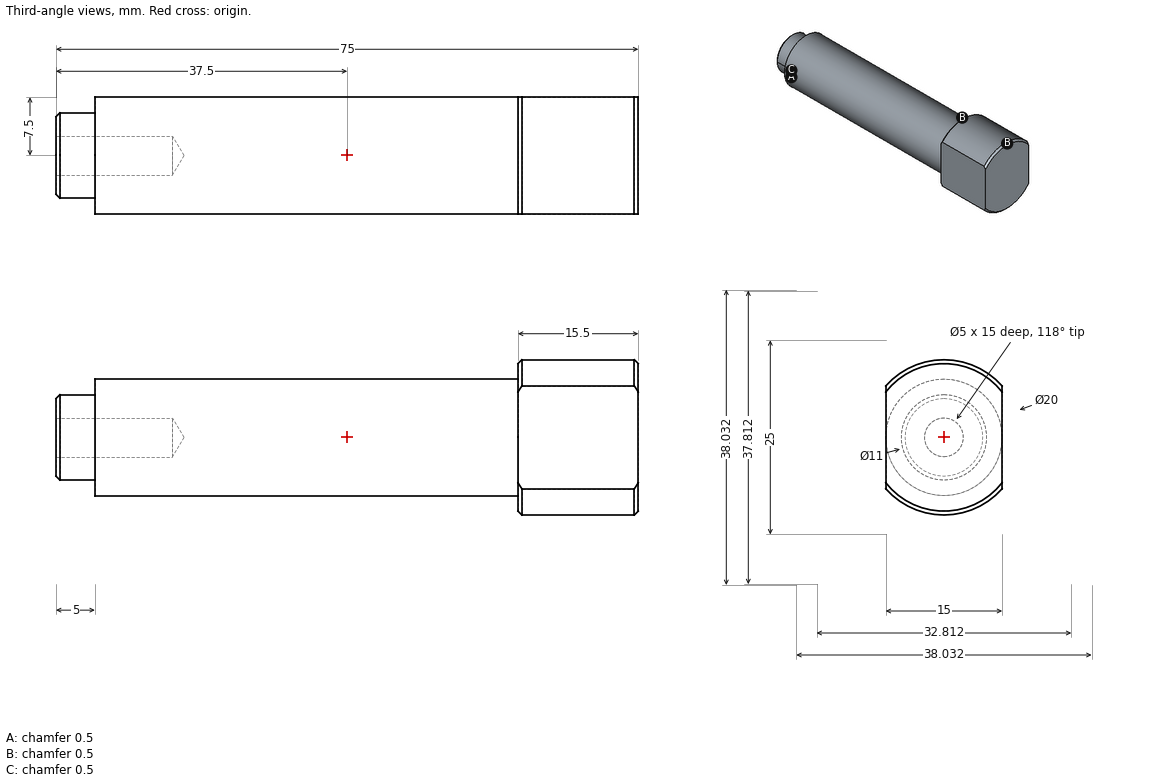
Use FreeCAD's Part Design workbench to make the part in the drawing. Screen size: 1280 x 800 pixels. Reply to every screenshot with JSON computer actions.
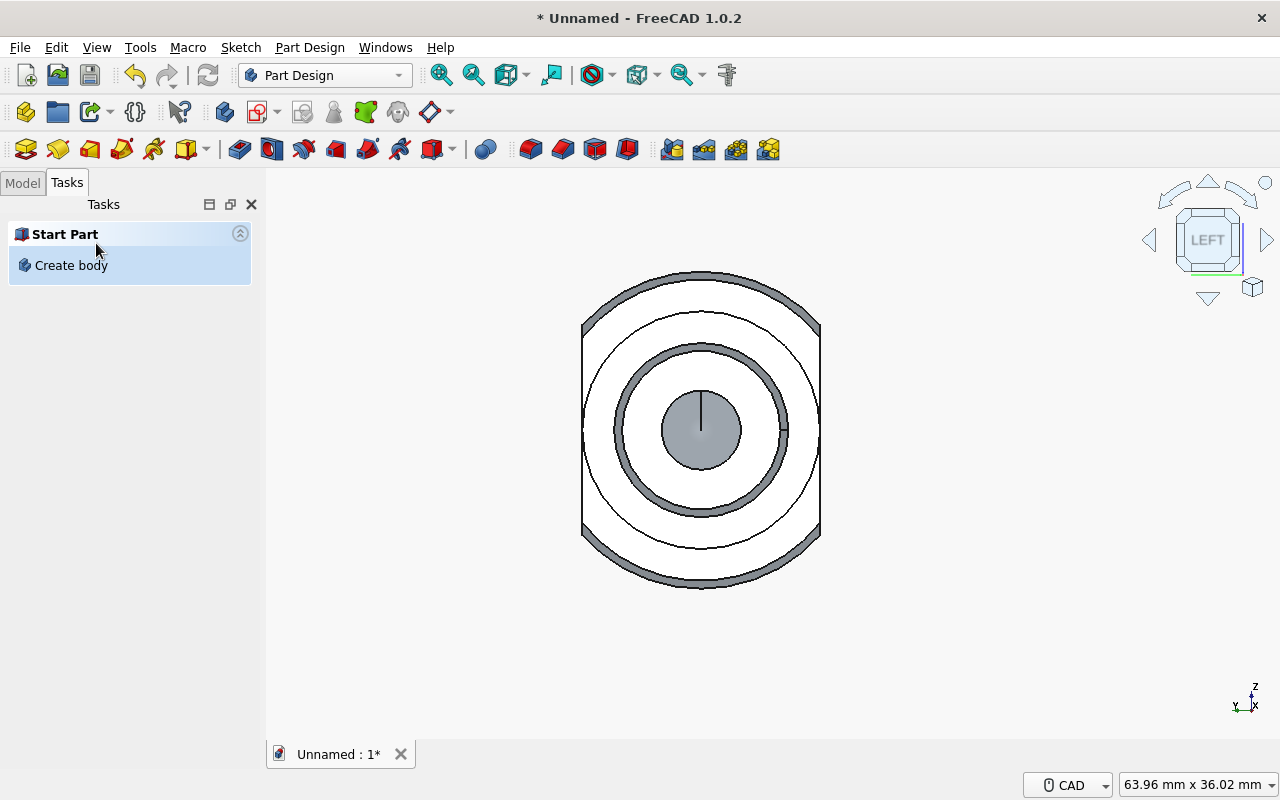
{"action": "key", "text": "0"}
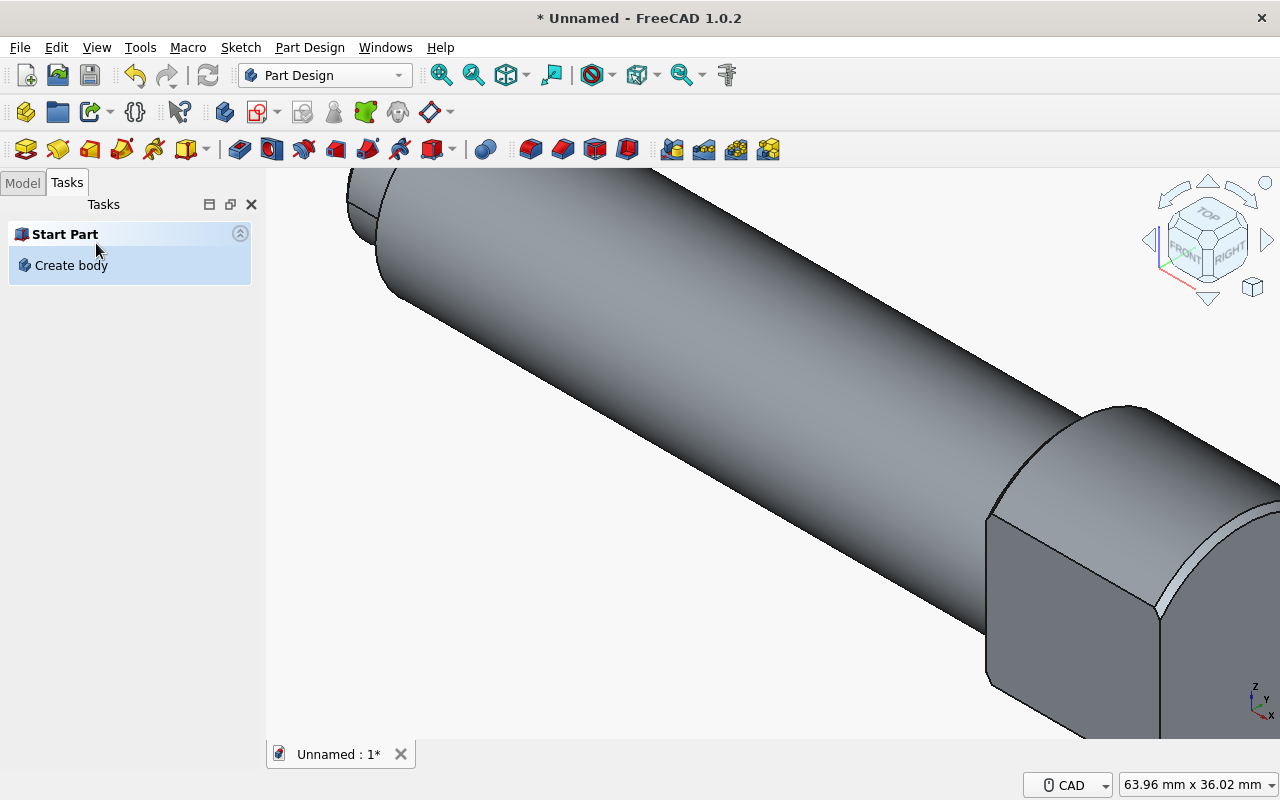
{"action": "left_click", "coordinate": [442, 76]}